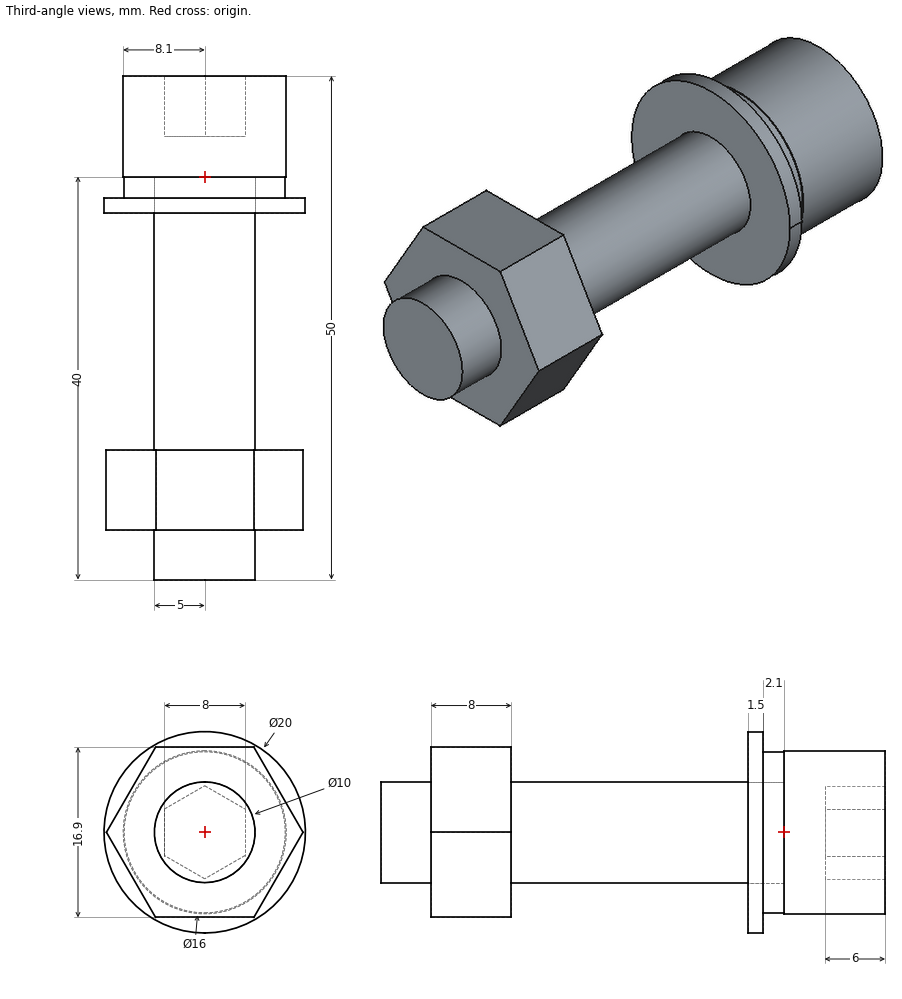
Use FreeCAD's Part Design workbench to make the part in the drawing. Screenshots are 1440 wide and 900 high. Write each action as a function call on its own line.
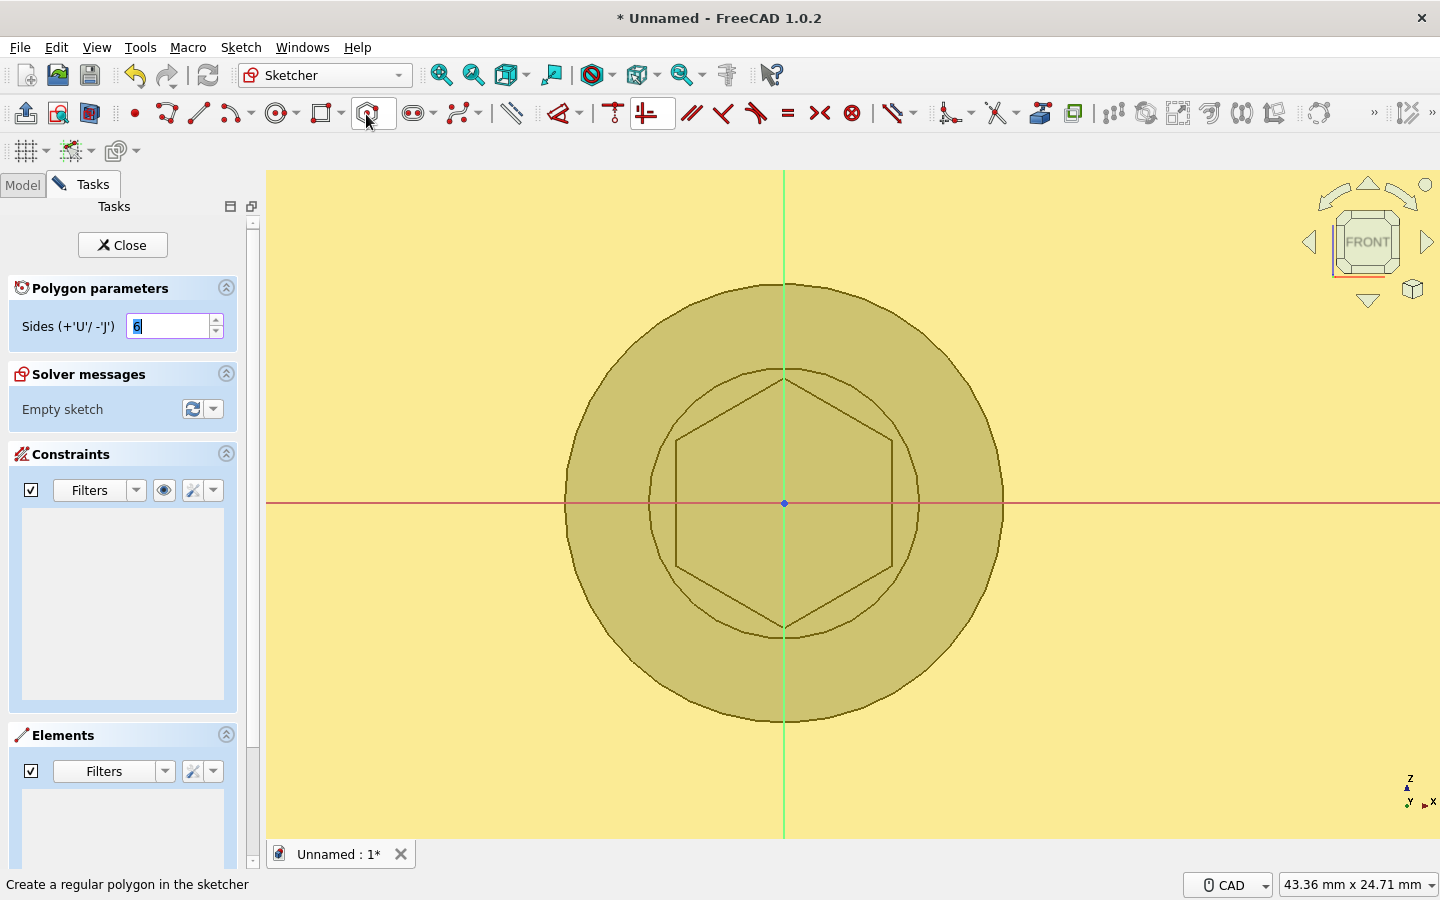
click(784, 503)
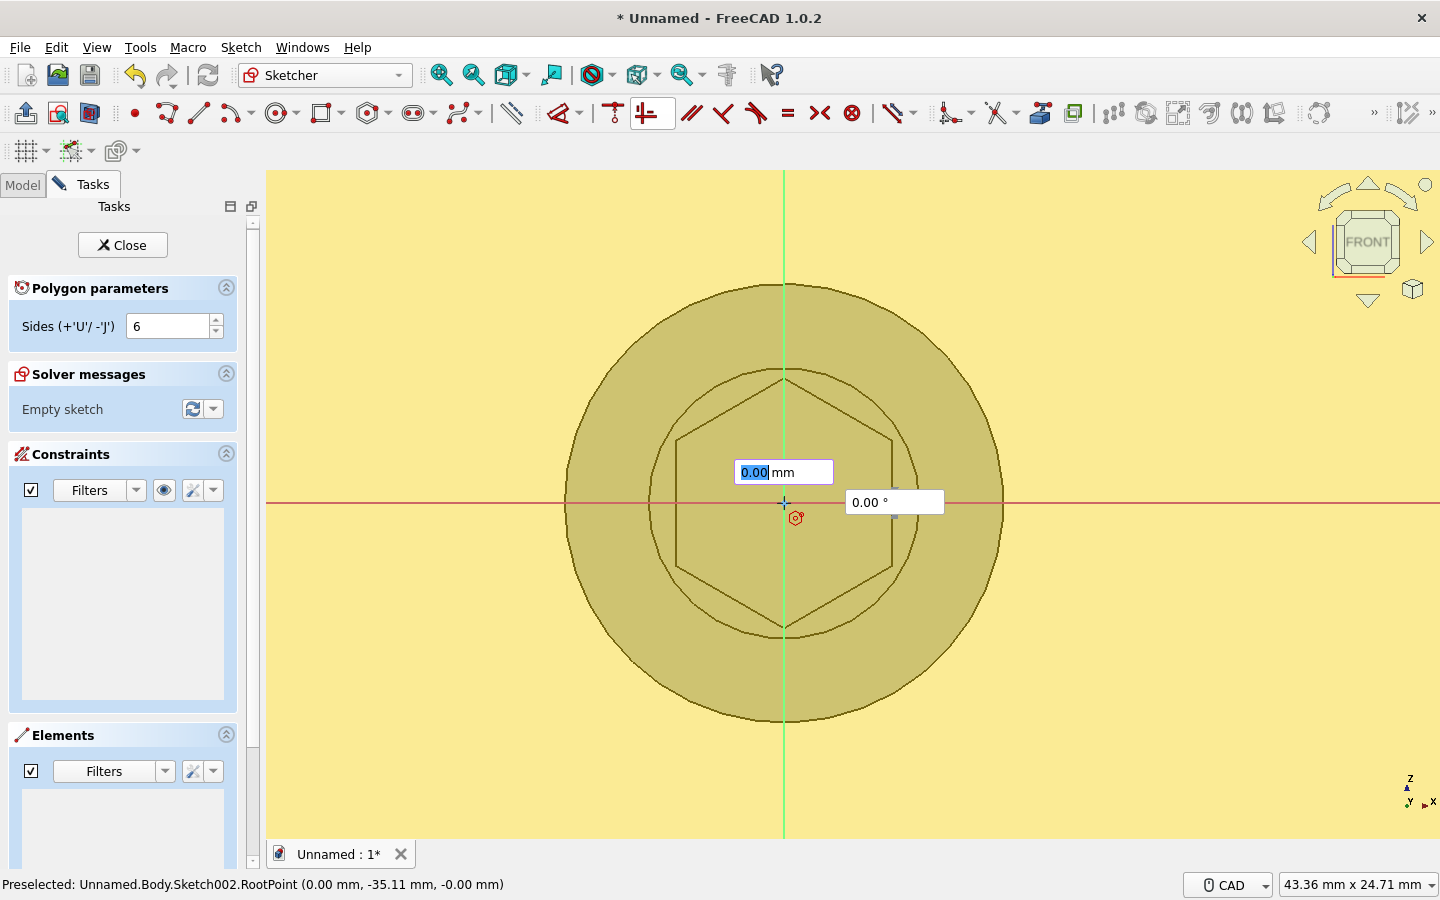
click(1048, 503)
right_click(1048, 503)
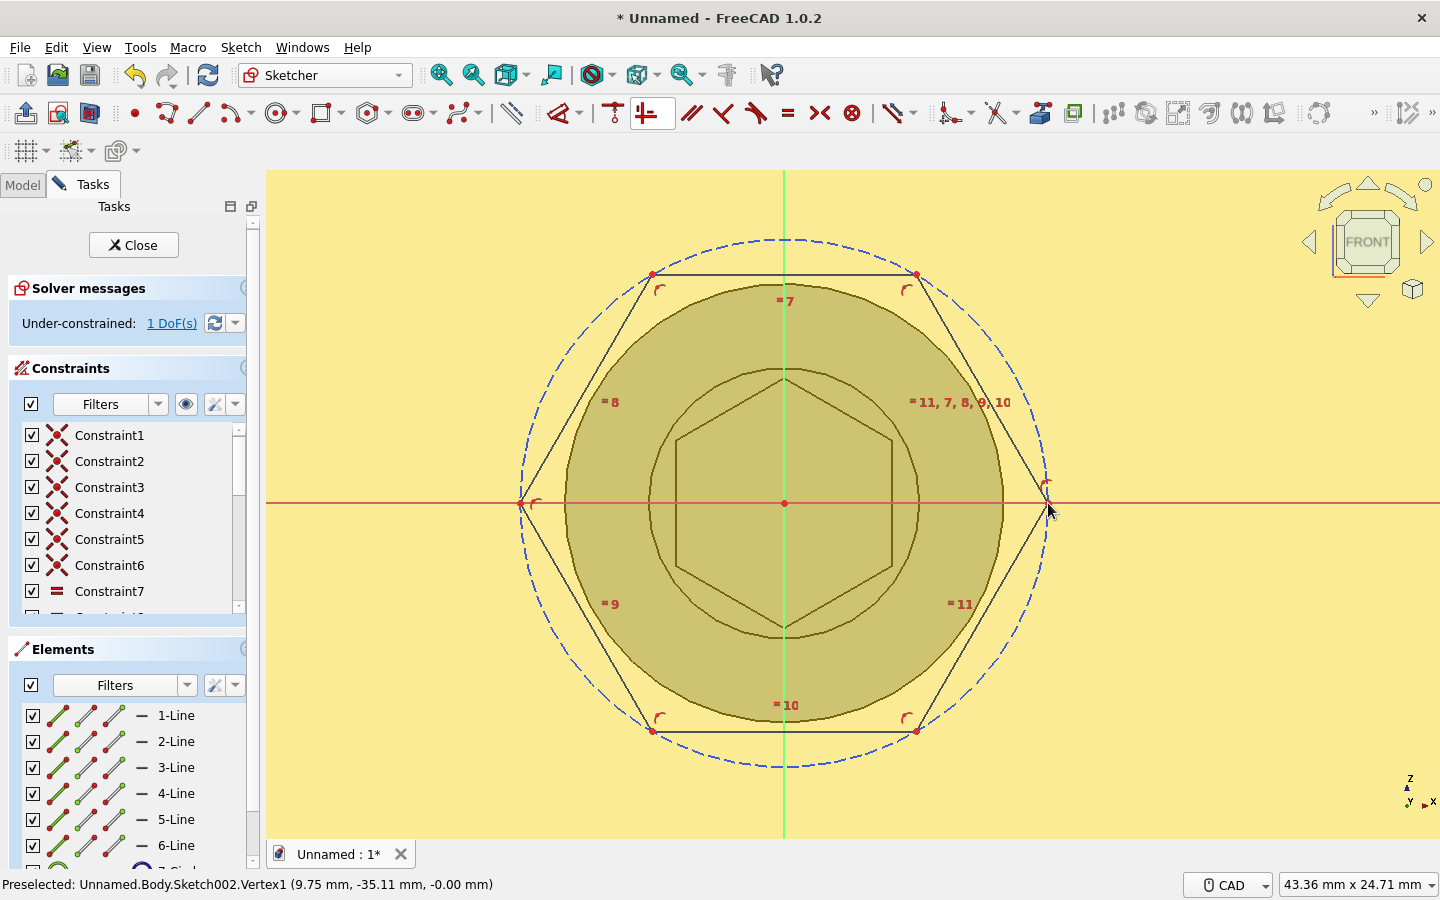
click(276, 114)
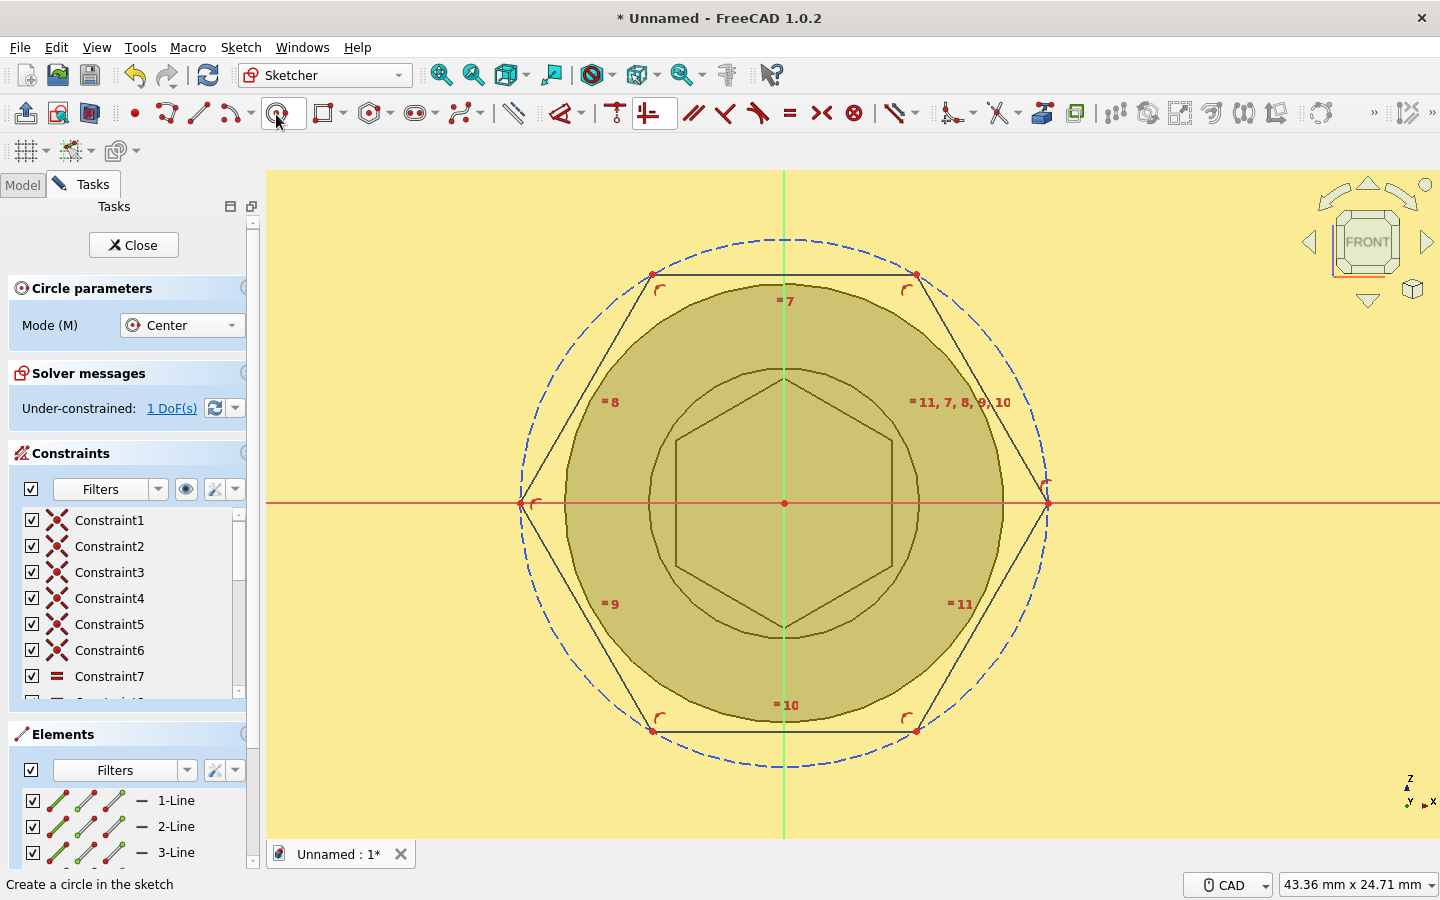
click(784, 503)
move(880, 408)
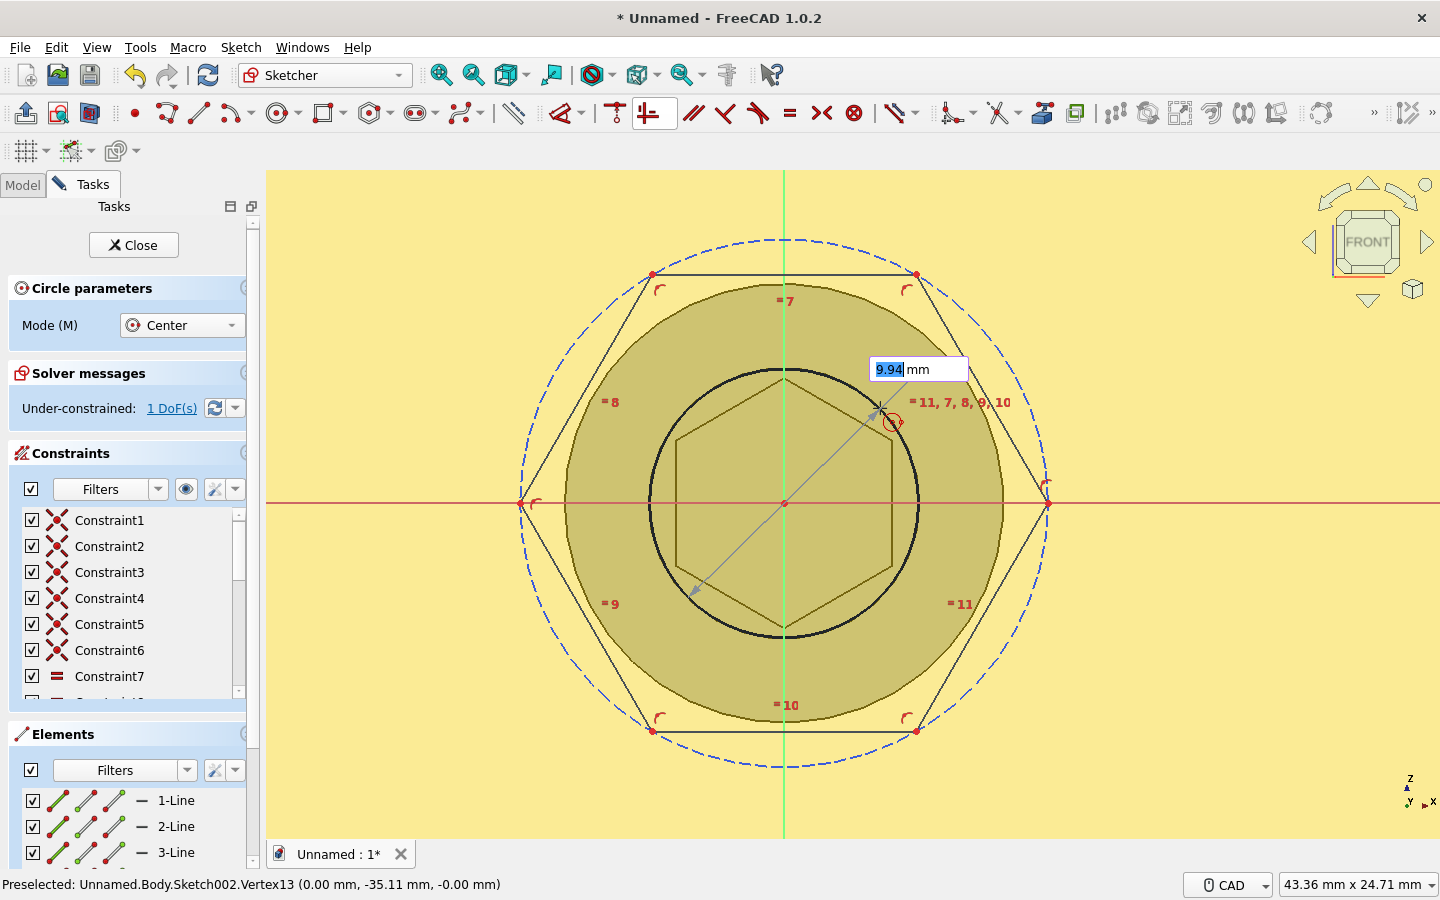
text(10)
key(Return)
key(Escape)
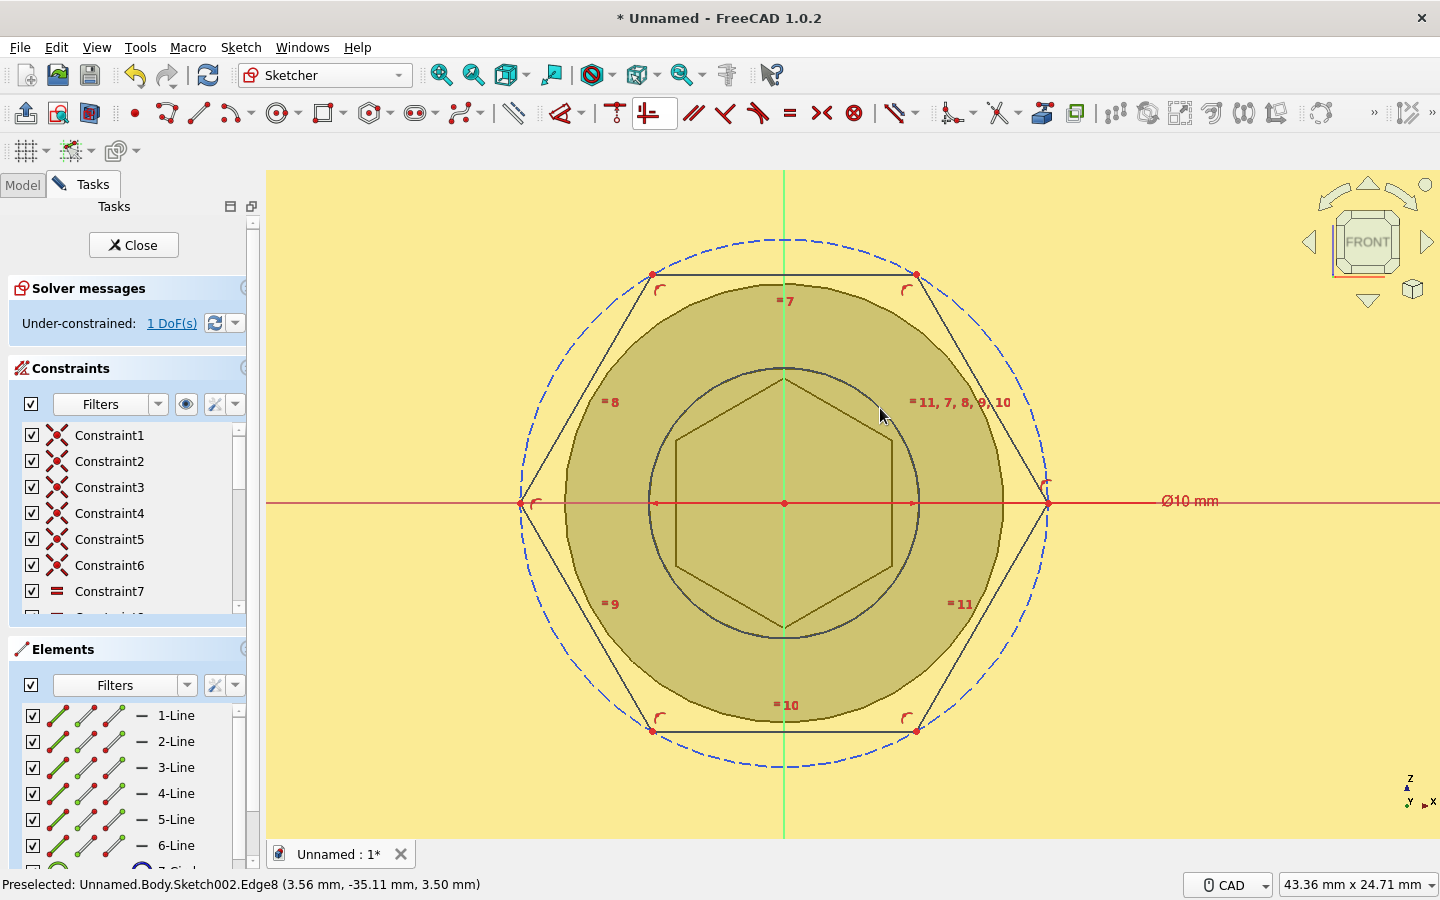
click(560, 114)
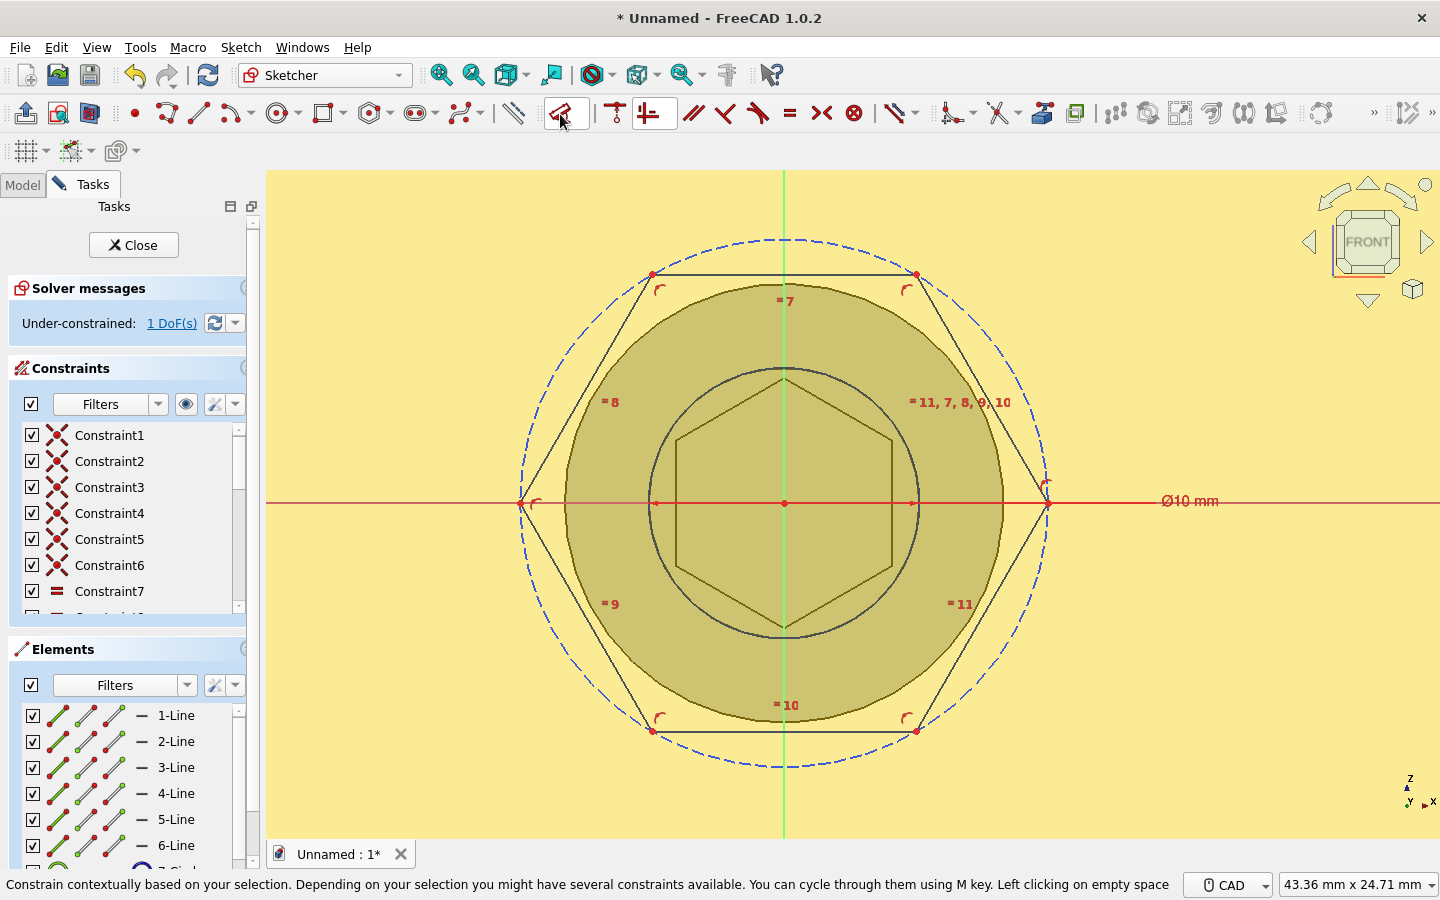
click(652, 732)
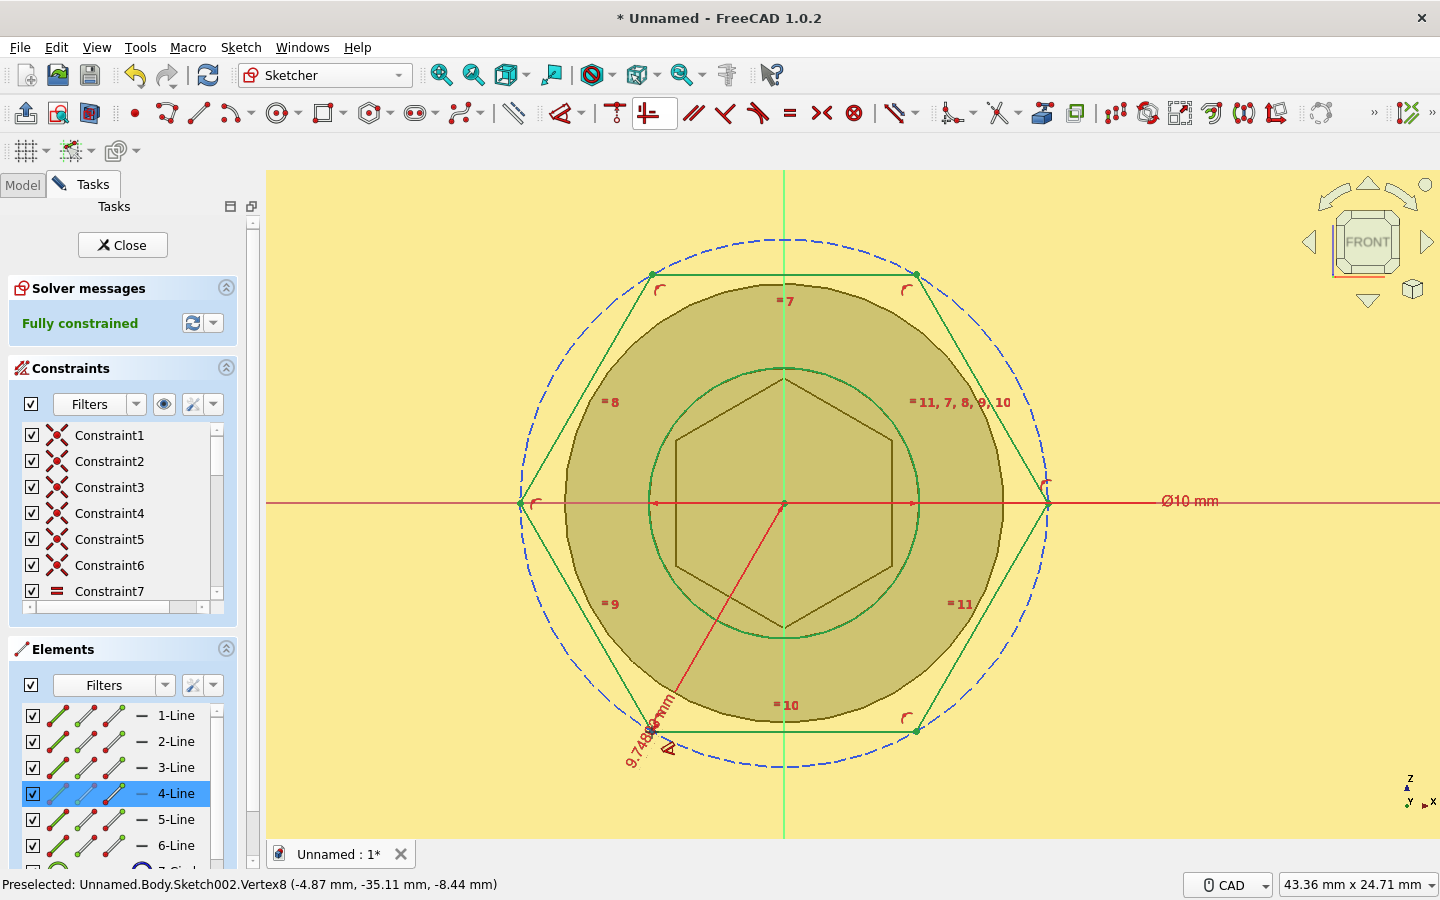
click(916, 275)
click(950, 398)